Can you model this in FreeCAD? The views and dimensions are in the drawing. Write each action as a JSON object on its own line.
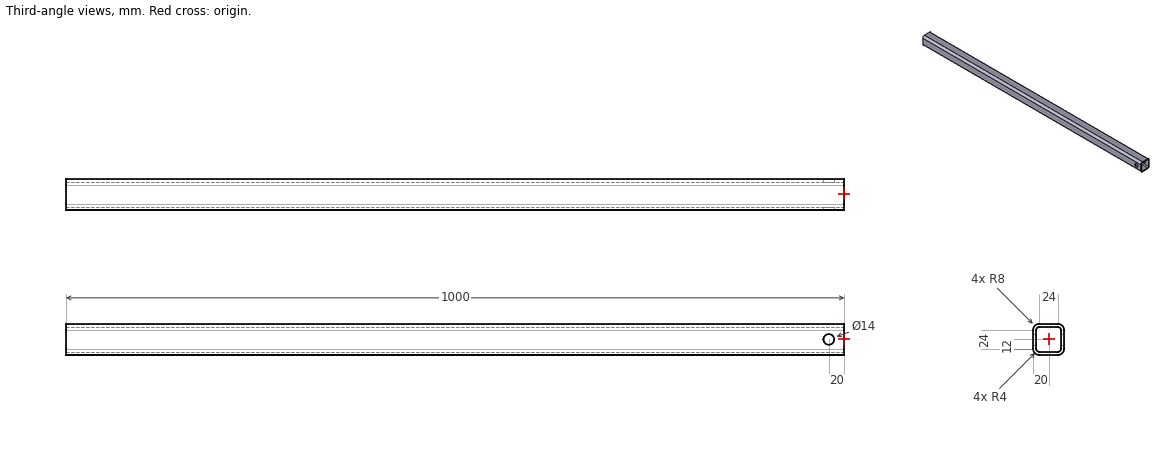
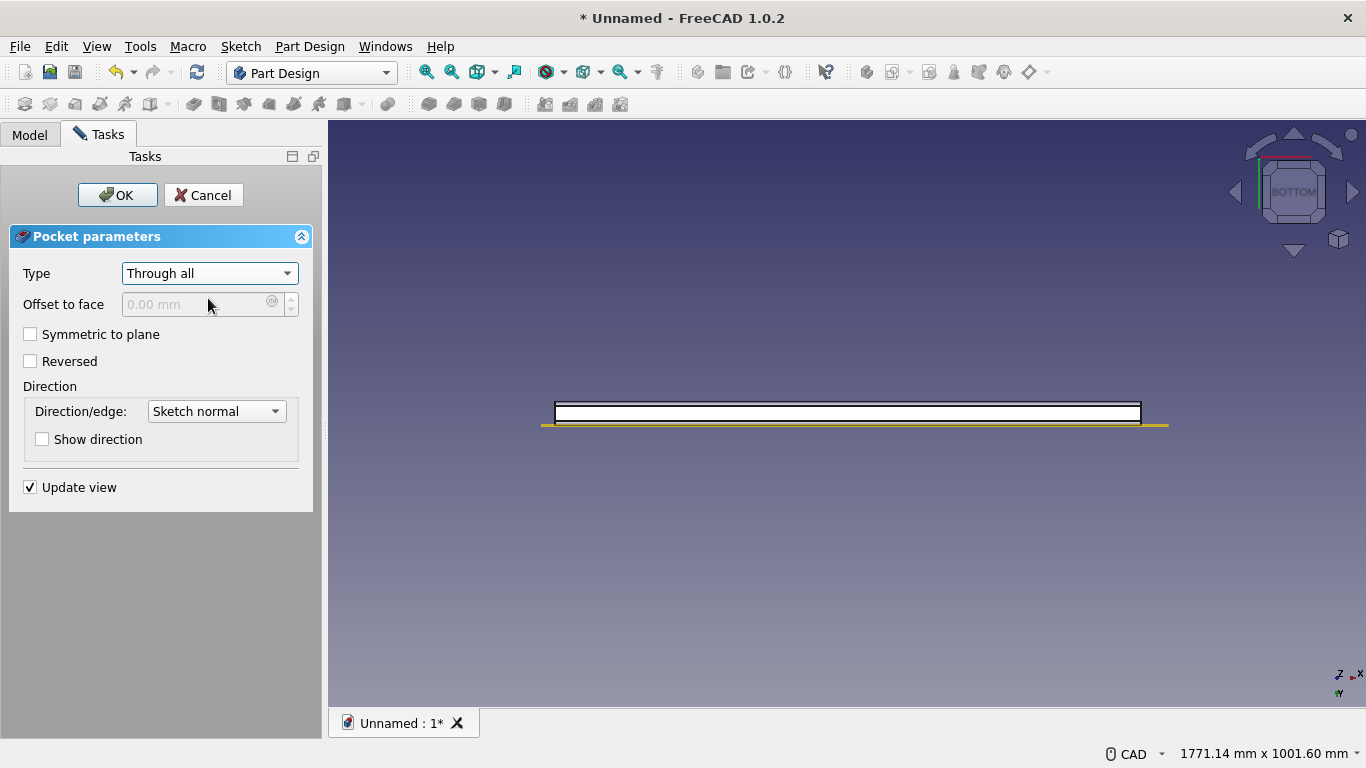
{"action": "left_click", "coordinate": [31, 361]}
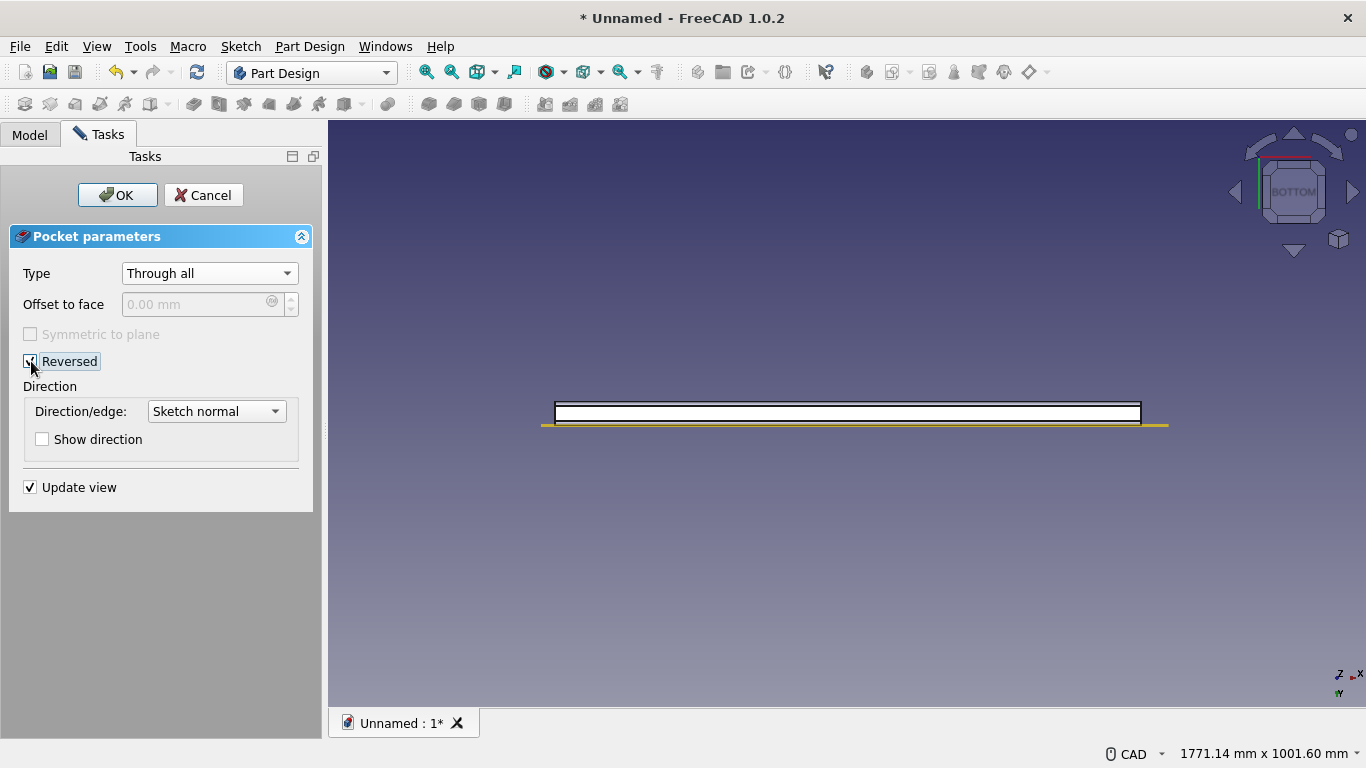
{"action": "left_click", "coordinate": [118, 195]}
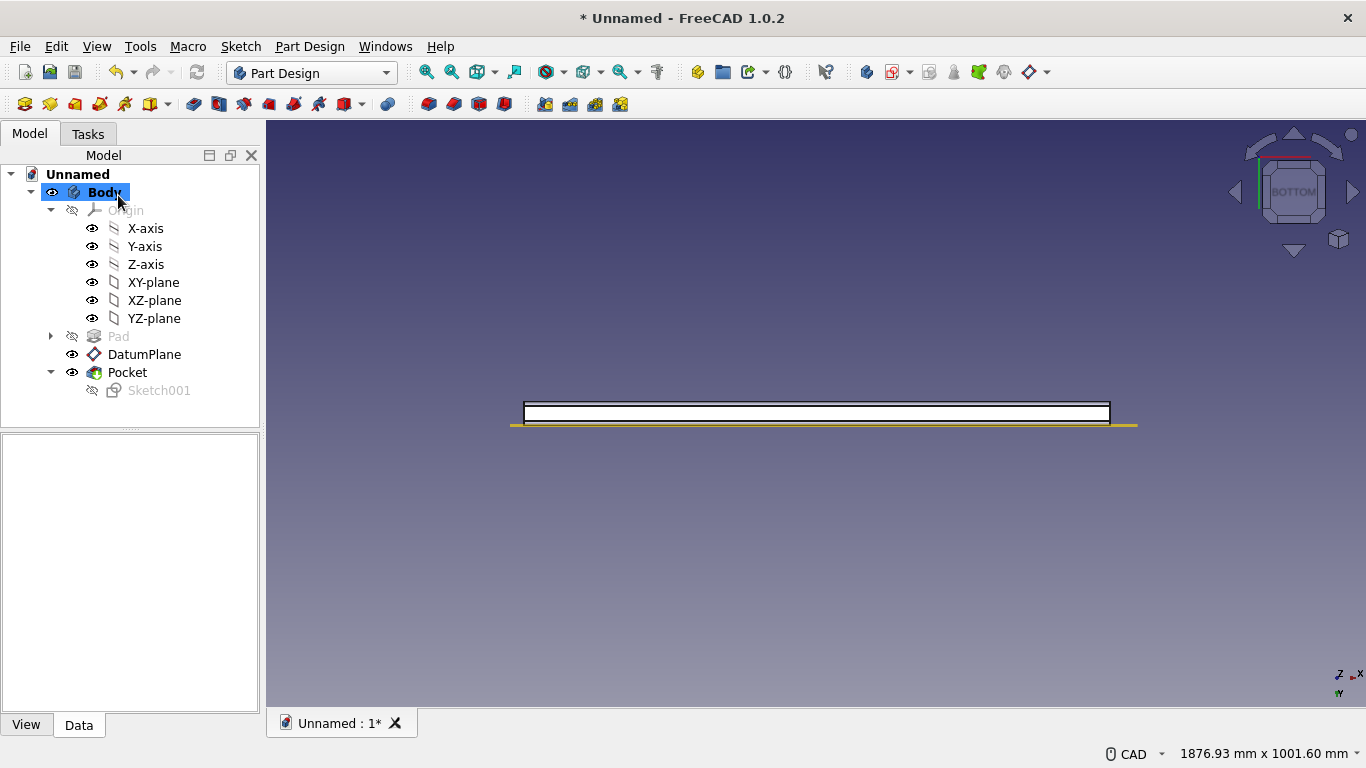
{"action": "left_click", "coordinate": [117, 354]}
{"action": "key", "text": "space"}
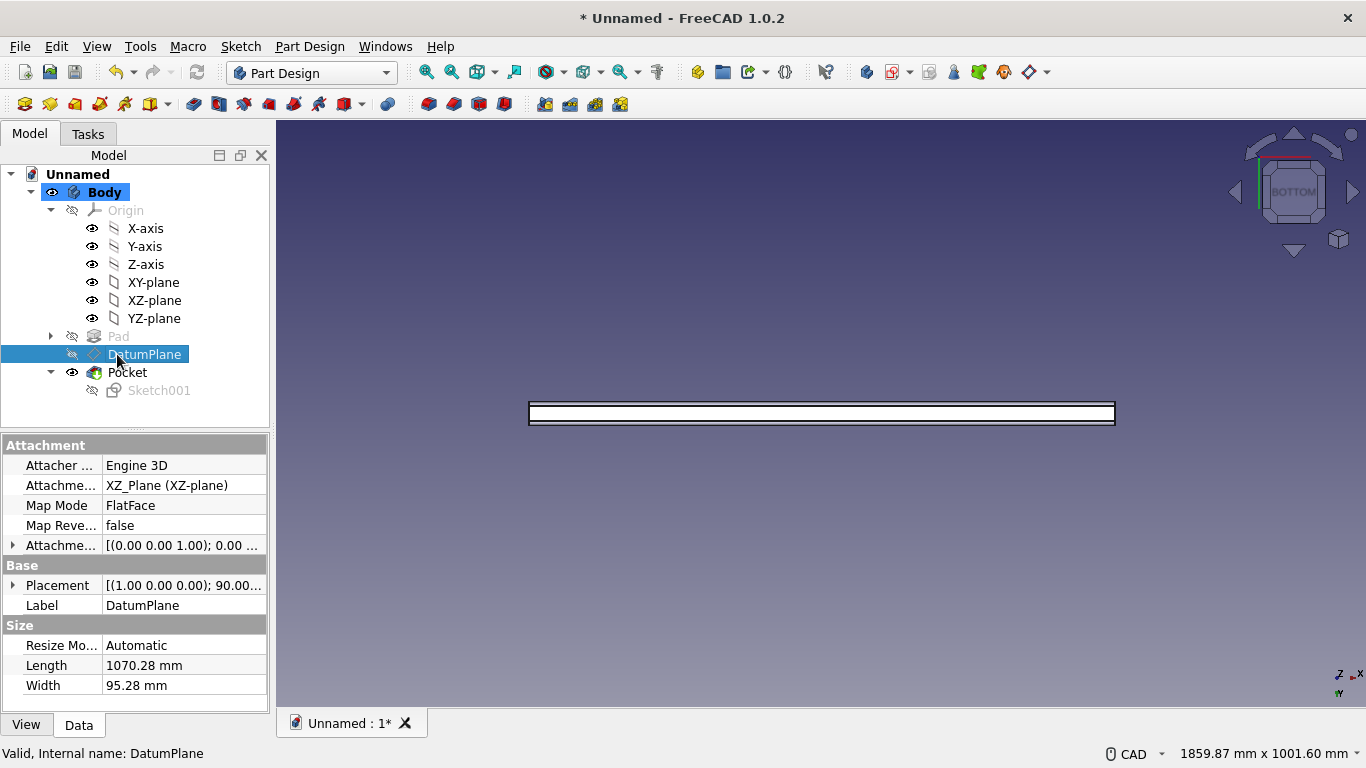
{"action": "key", "text": "0"}